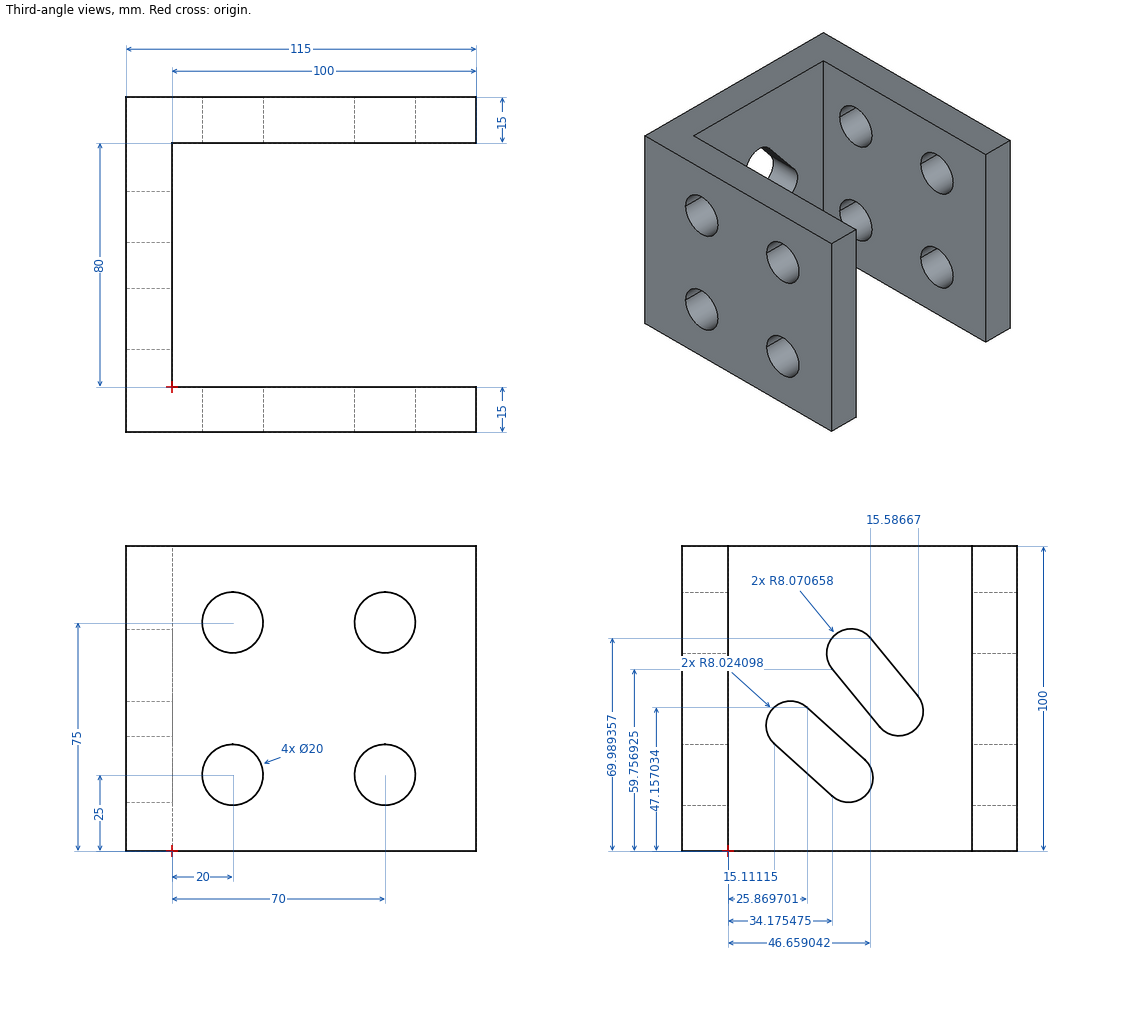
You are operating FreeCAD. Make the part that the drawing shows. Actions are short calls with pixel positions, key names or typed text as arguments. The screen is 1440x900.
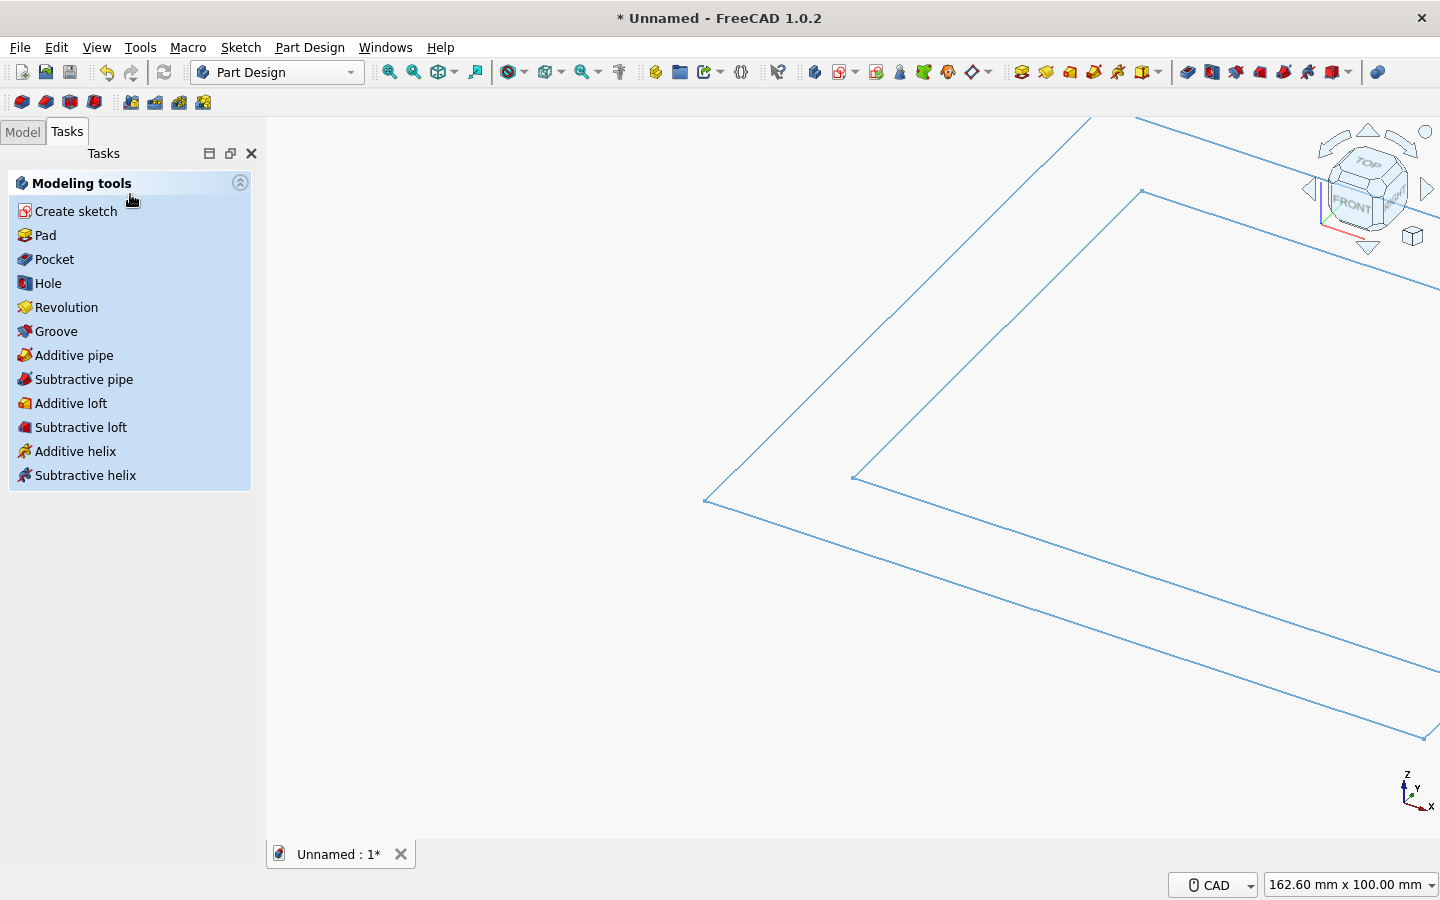
click(1022, 72)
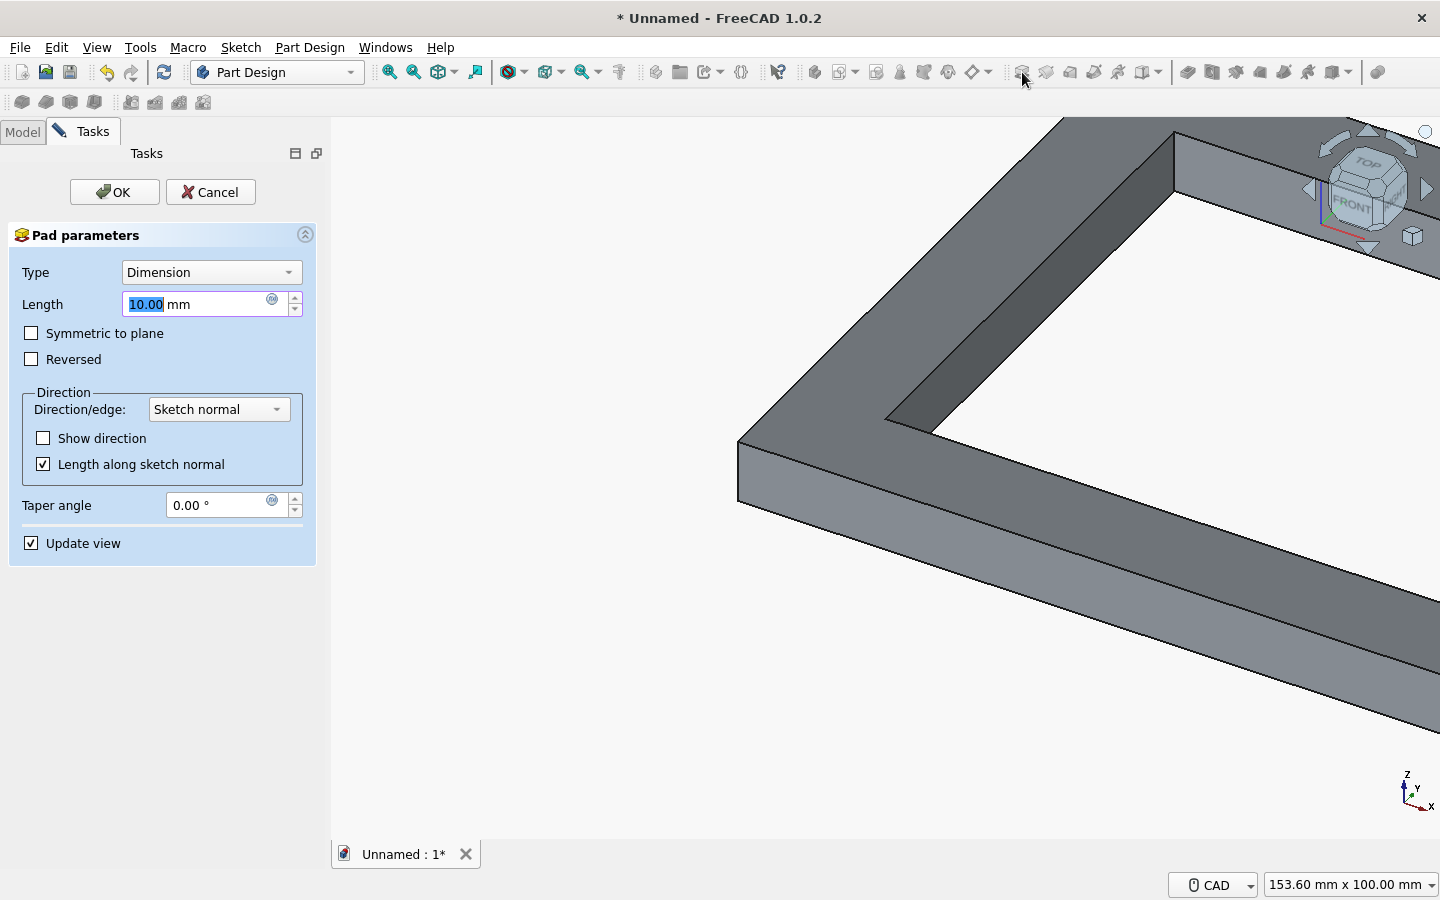
text(100)
key(Tab)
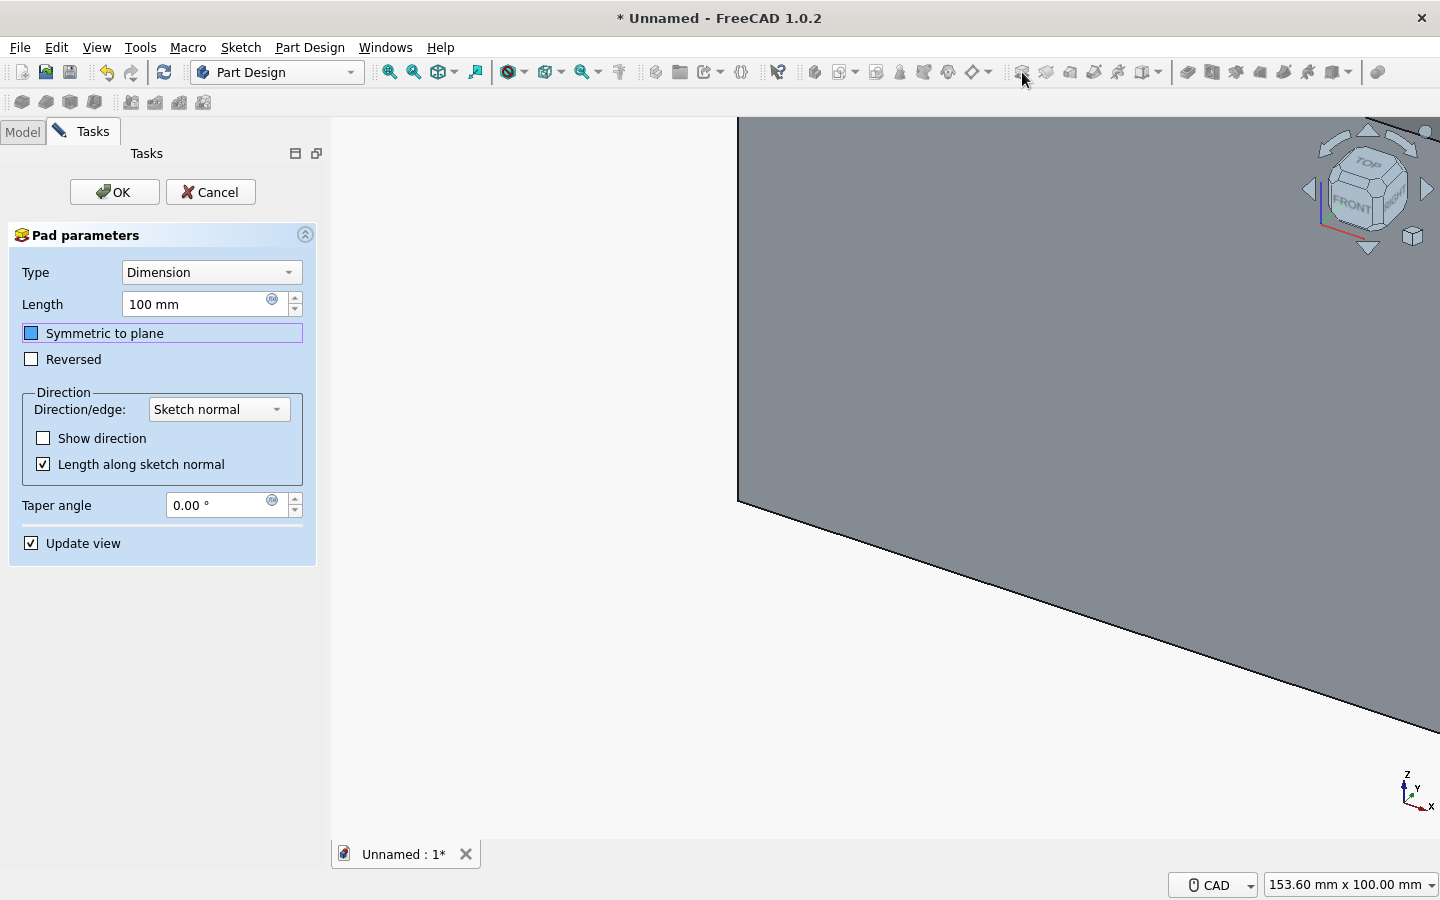
click(115, 192)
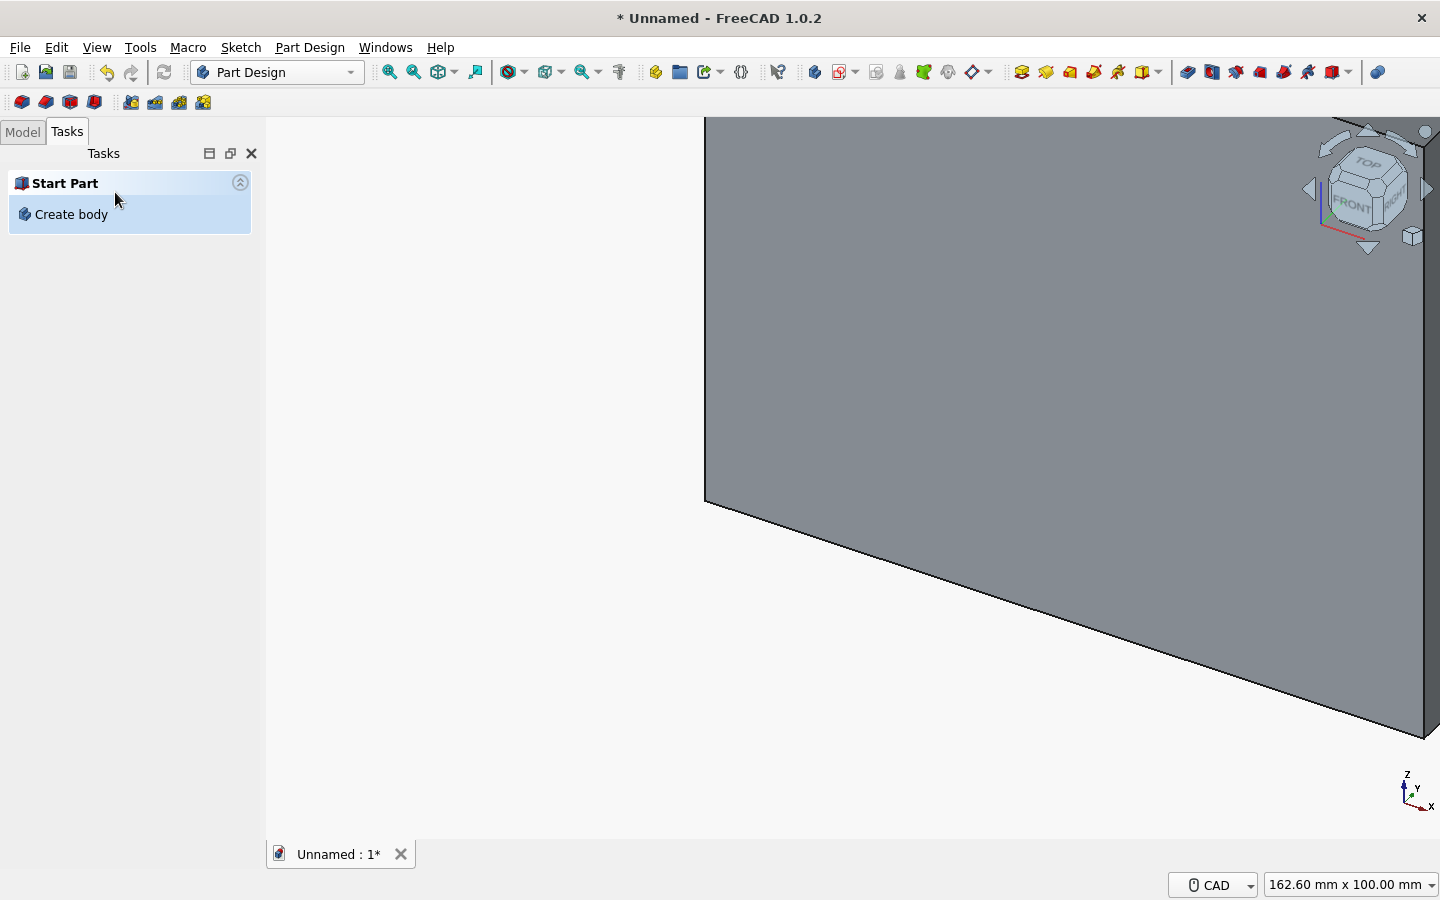
key(v)
key(f)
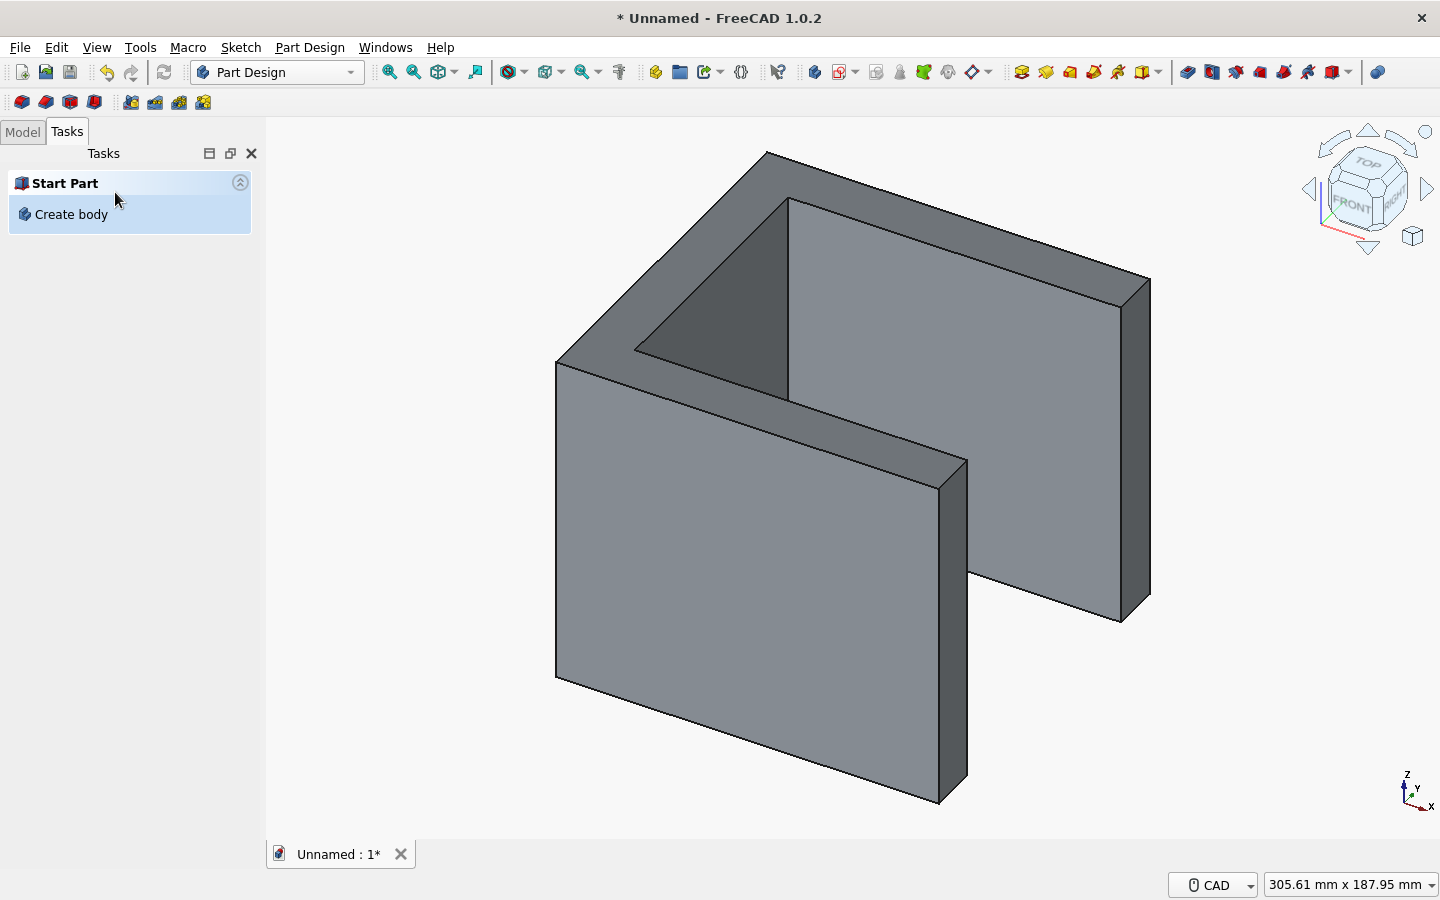
key(4)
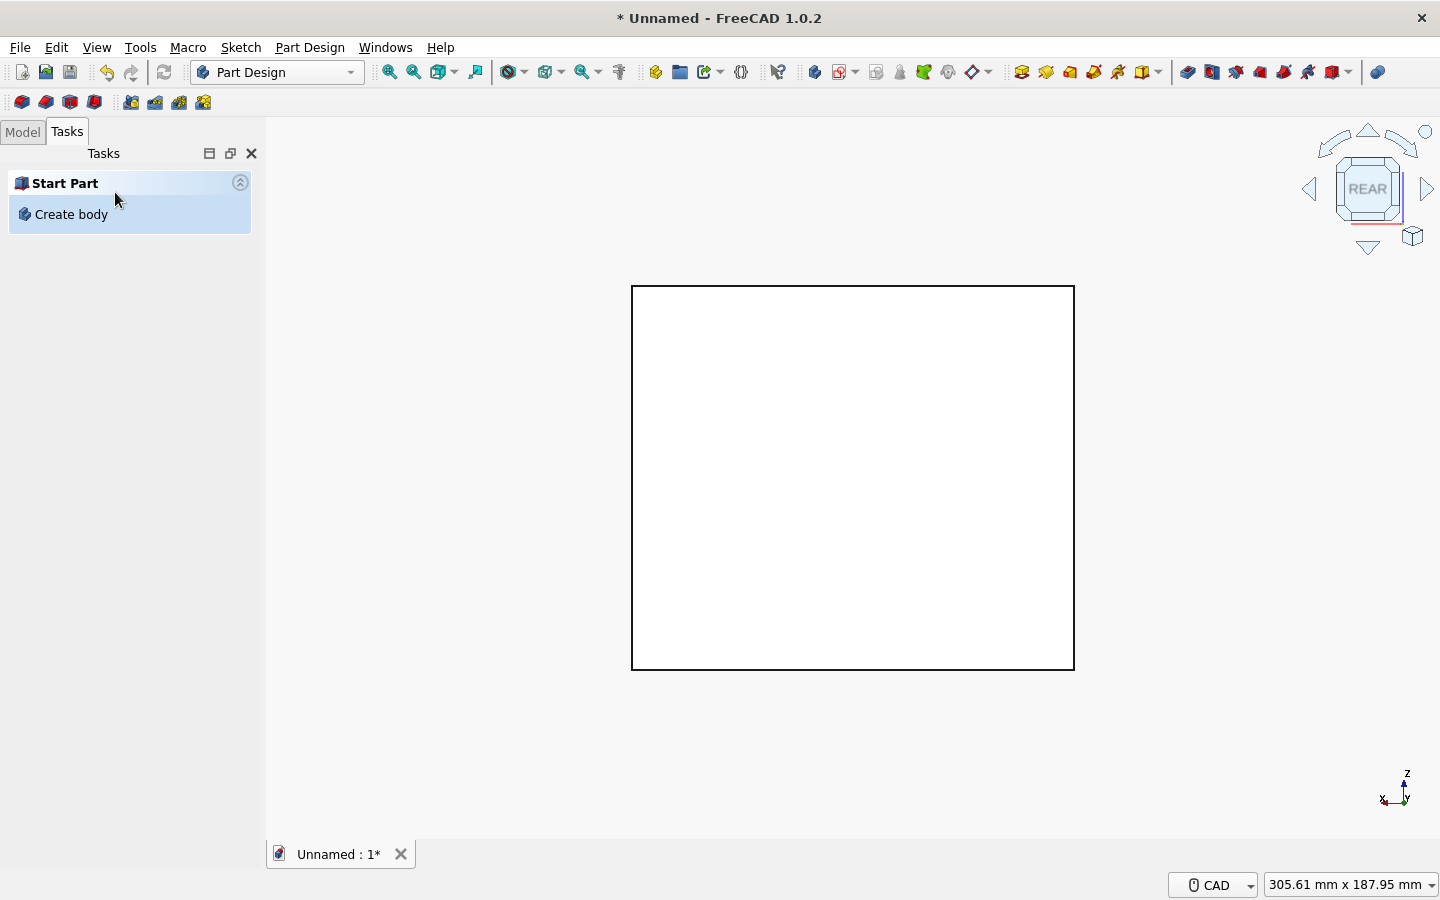
click(853, 477)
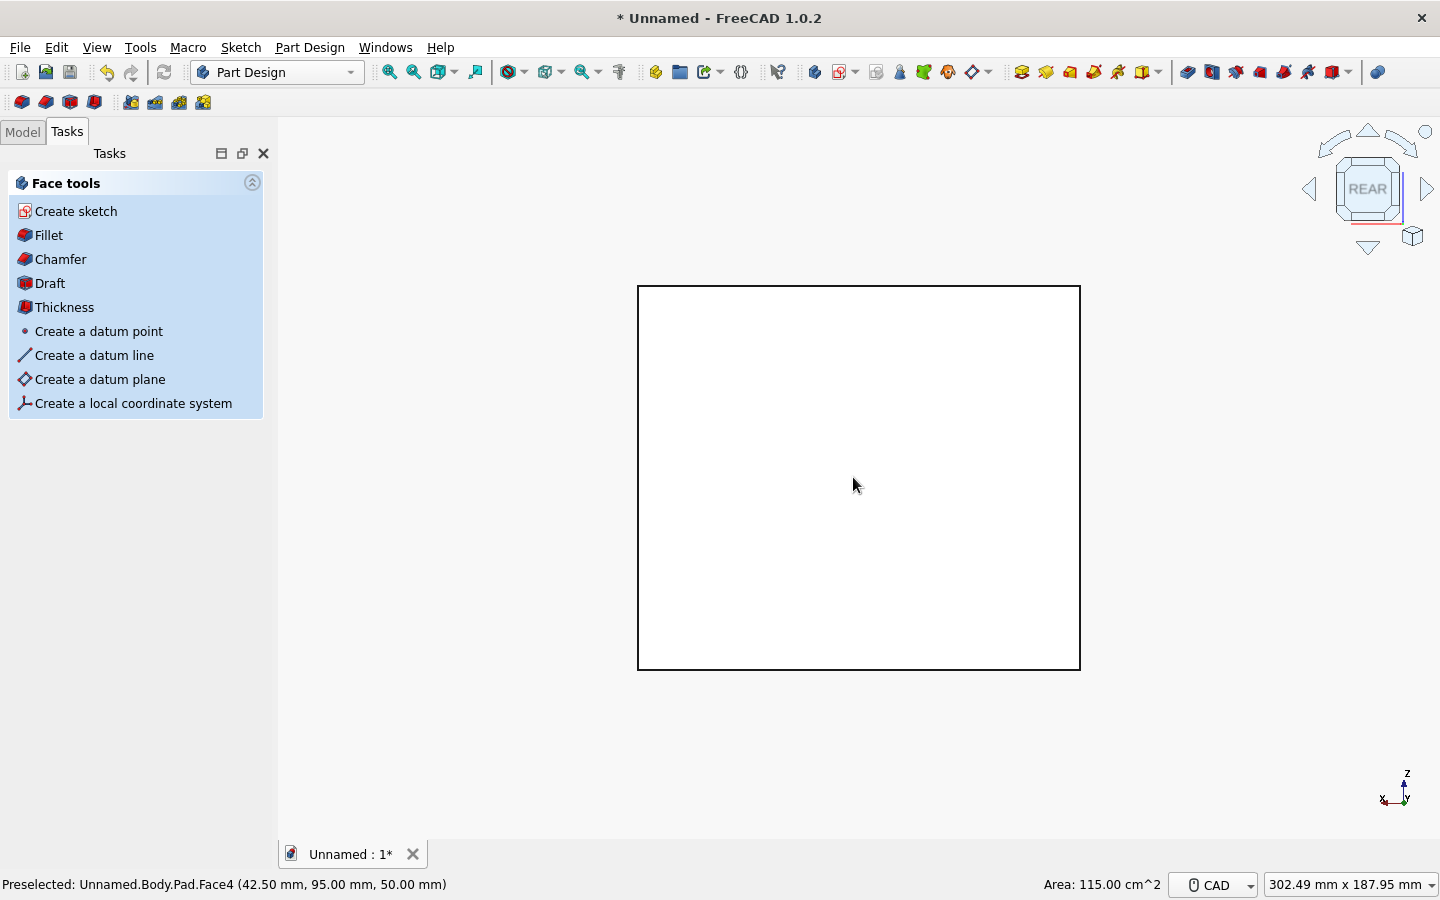
click(840, 72)